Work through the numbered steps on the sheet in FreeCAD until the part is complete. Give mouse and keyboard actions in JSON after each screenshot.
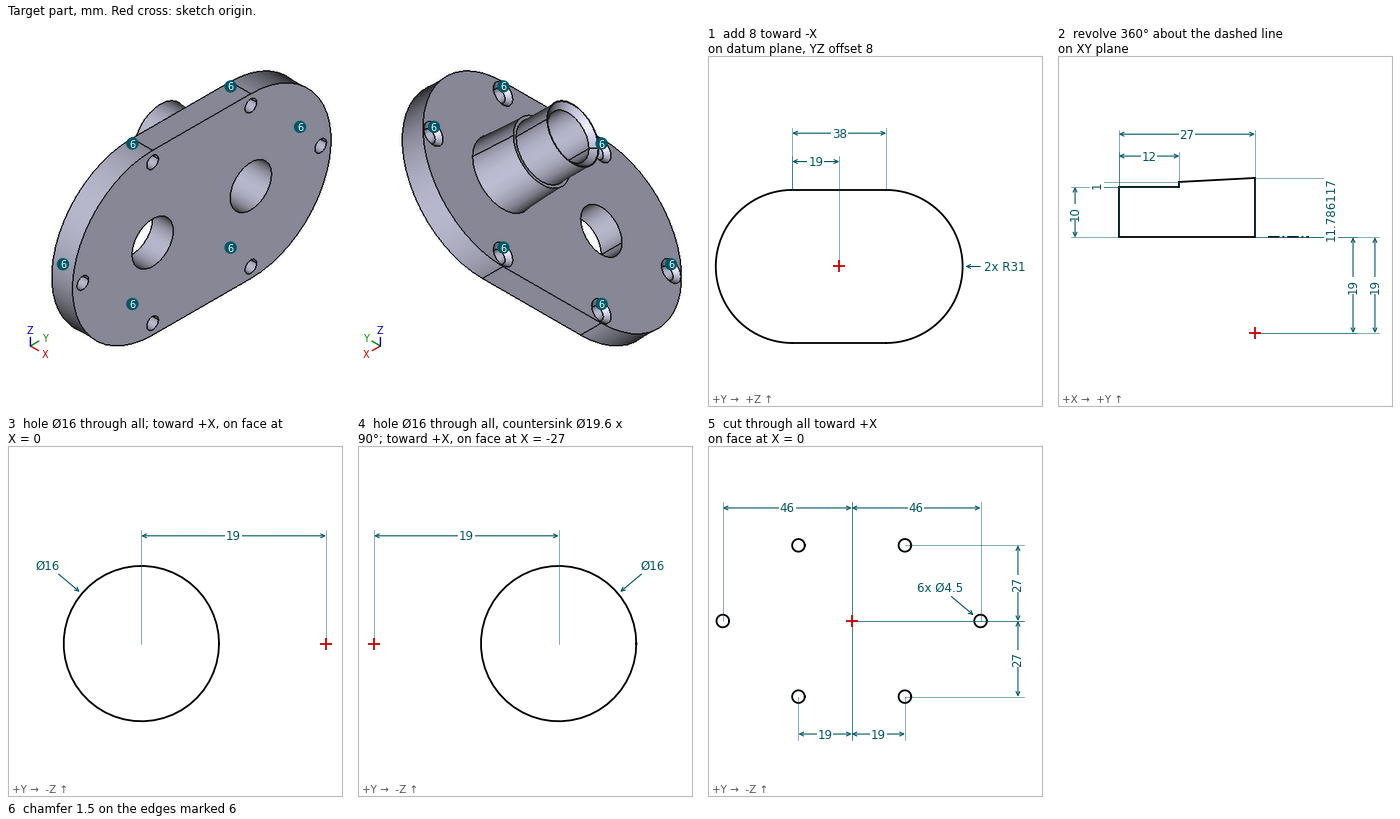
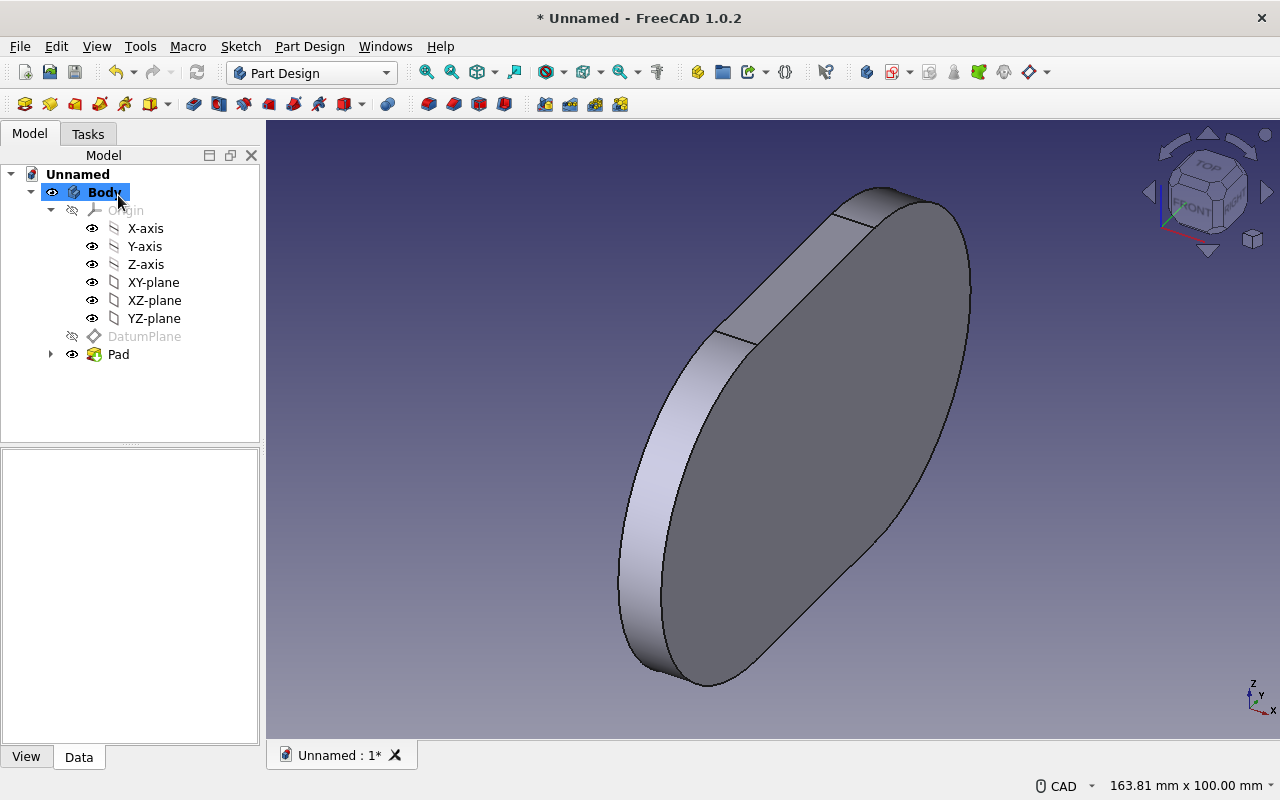
{"action": "key", "text": "v f"}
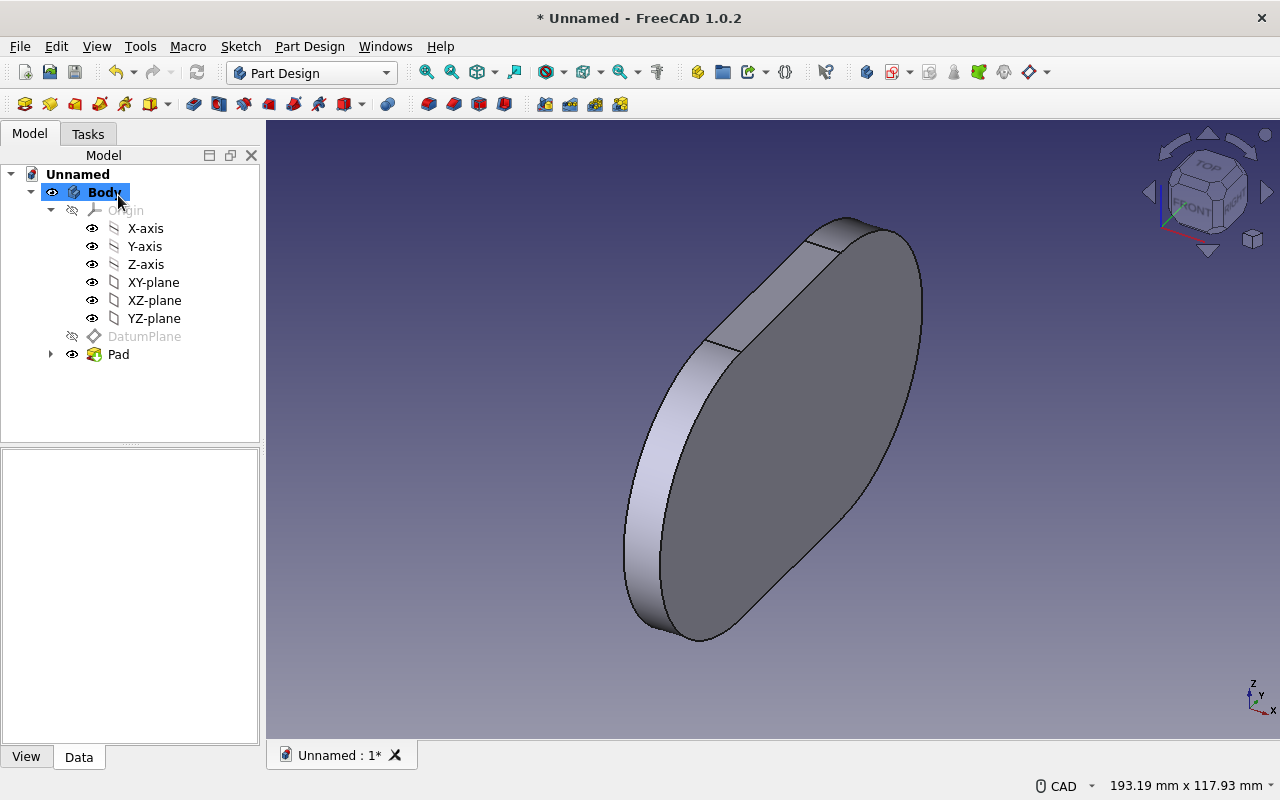
{"action": "left_click", "coordinate": [892, 72]}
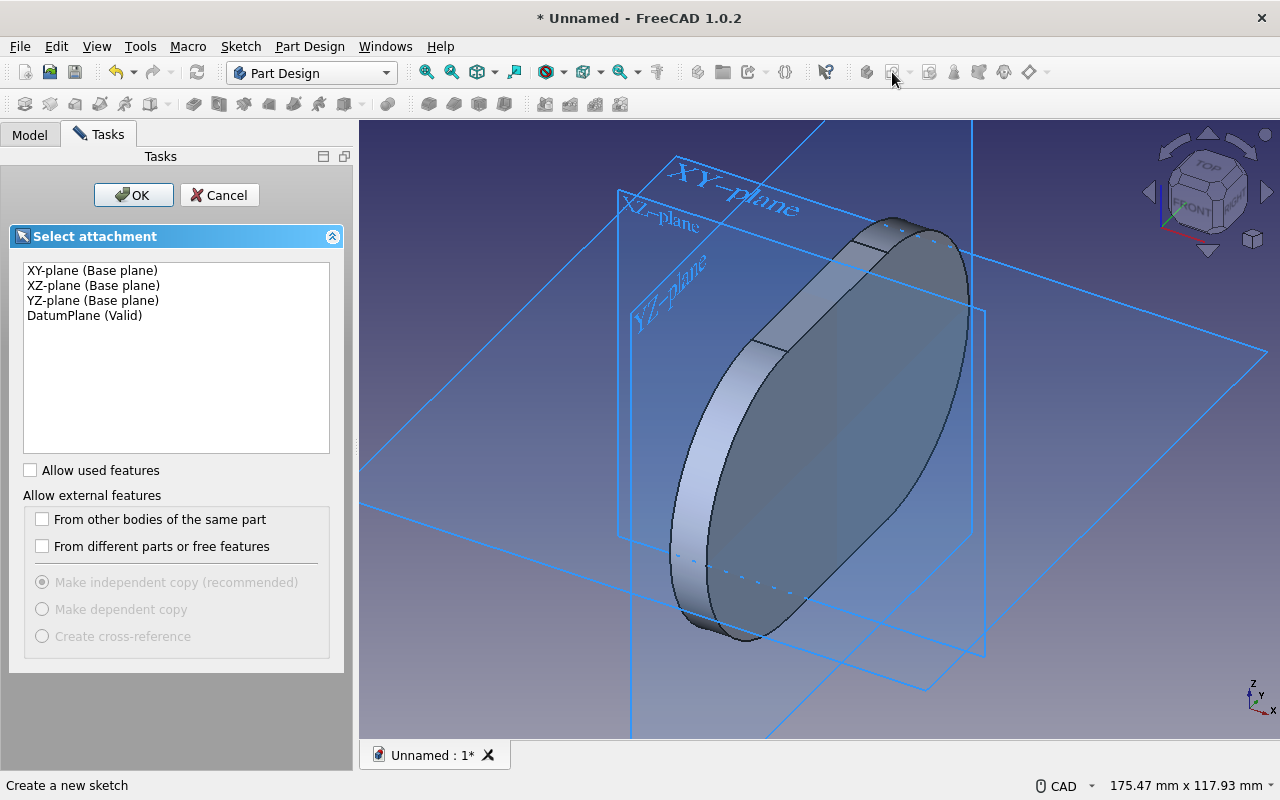
{"action": "left_click", "coordinate": [84, 270]}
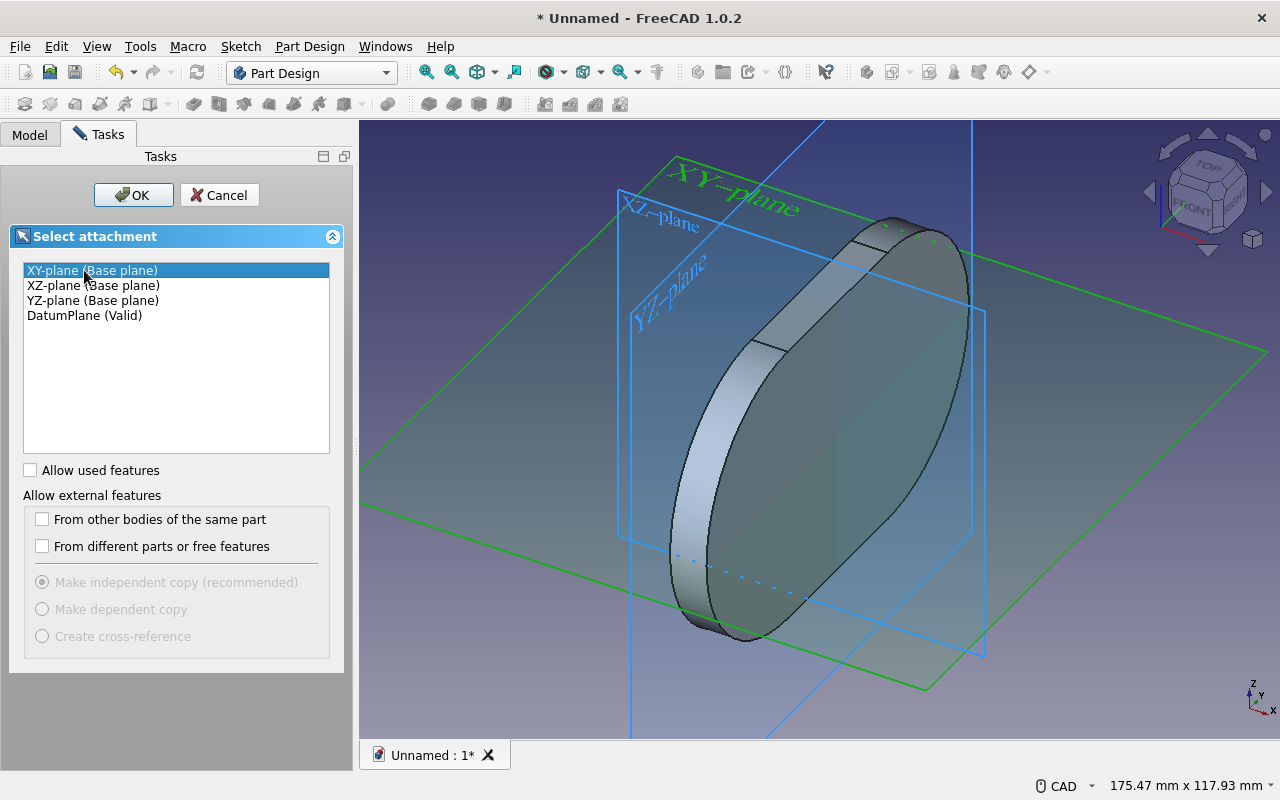
{"action": "left_click", "coordinate": [134, 195]}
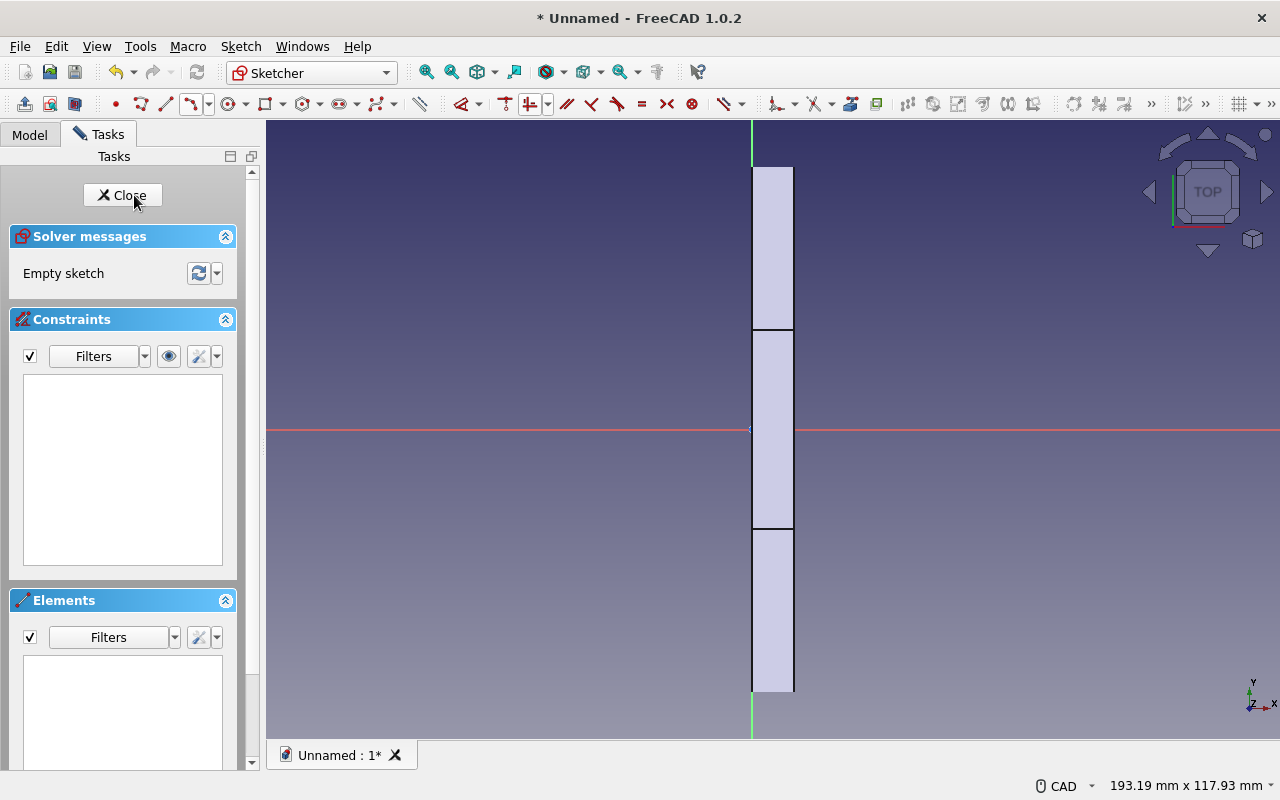
{"action": "key", "text": "q s"}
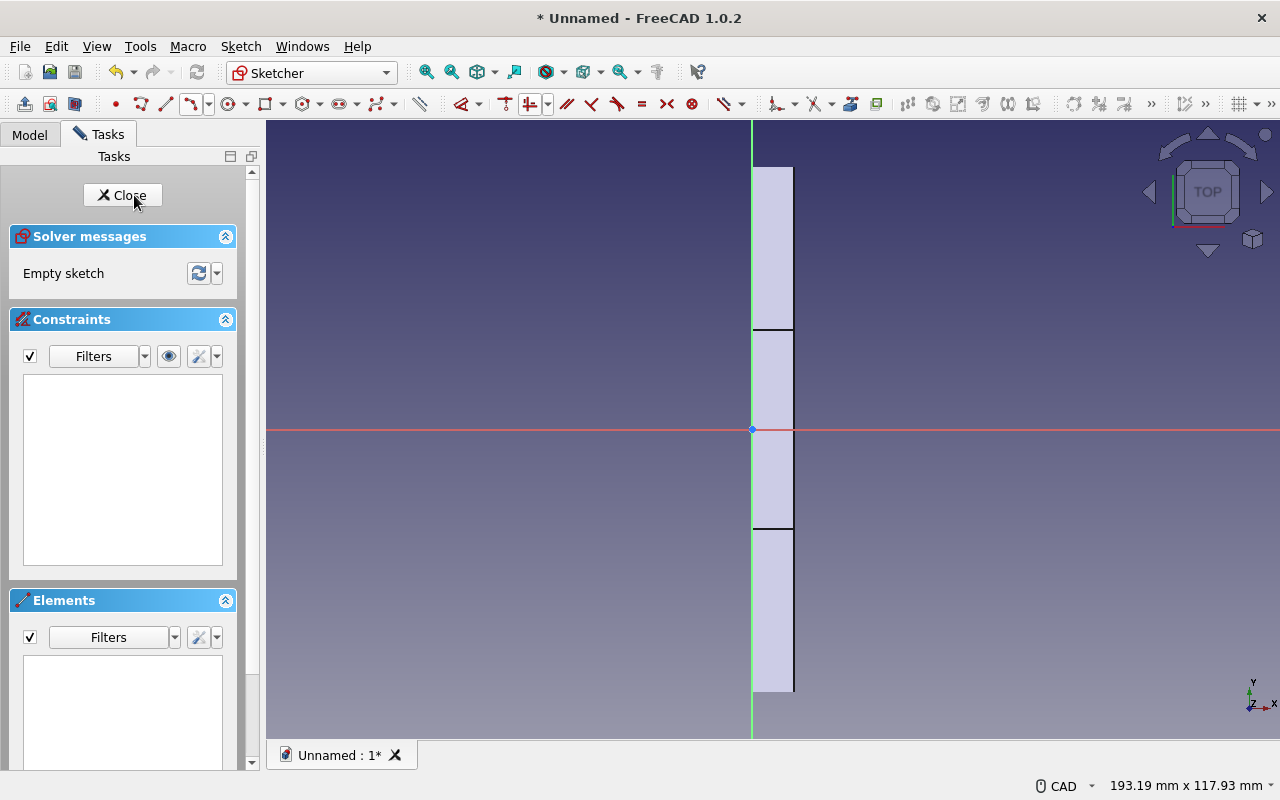
{"action": "scroll", "coordinate": [714, 283], "scroll_direction": "up", "scroll_amount": 4}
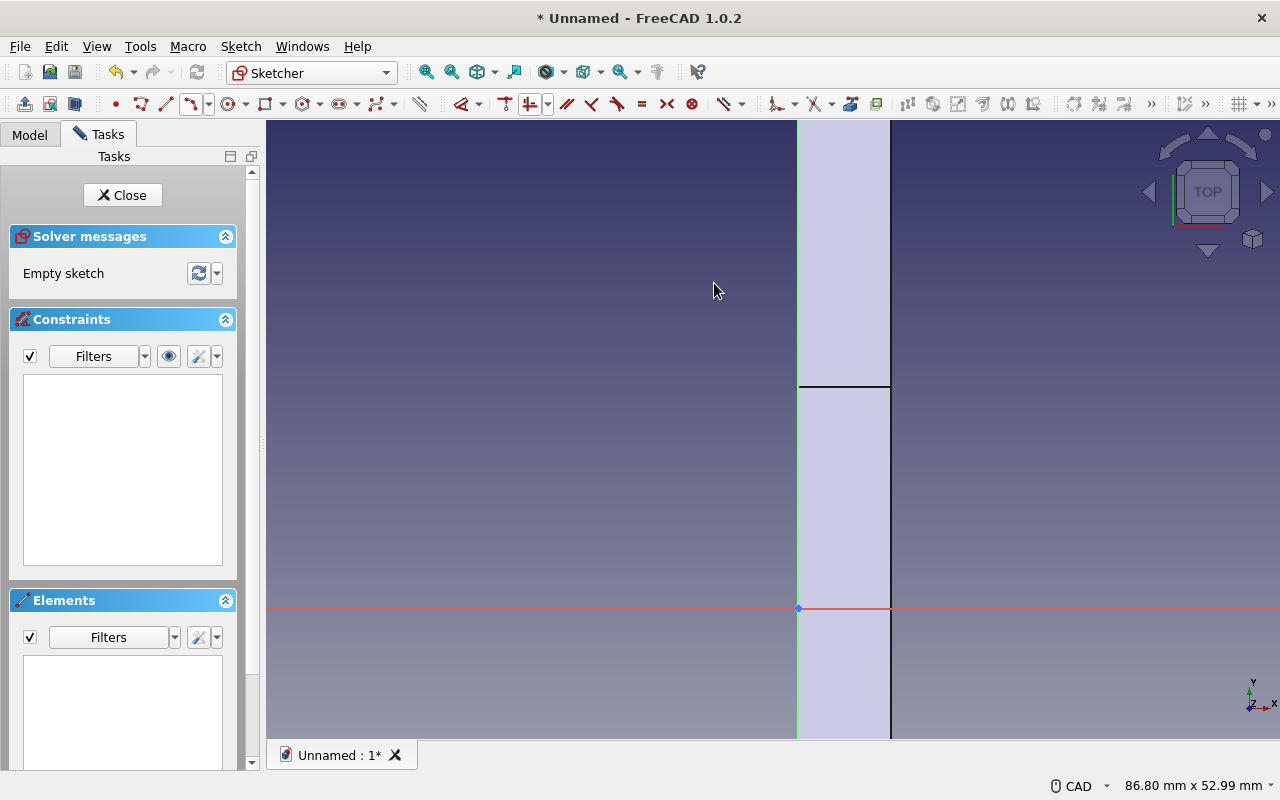
{"action": "key", "text": "g m"}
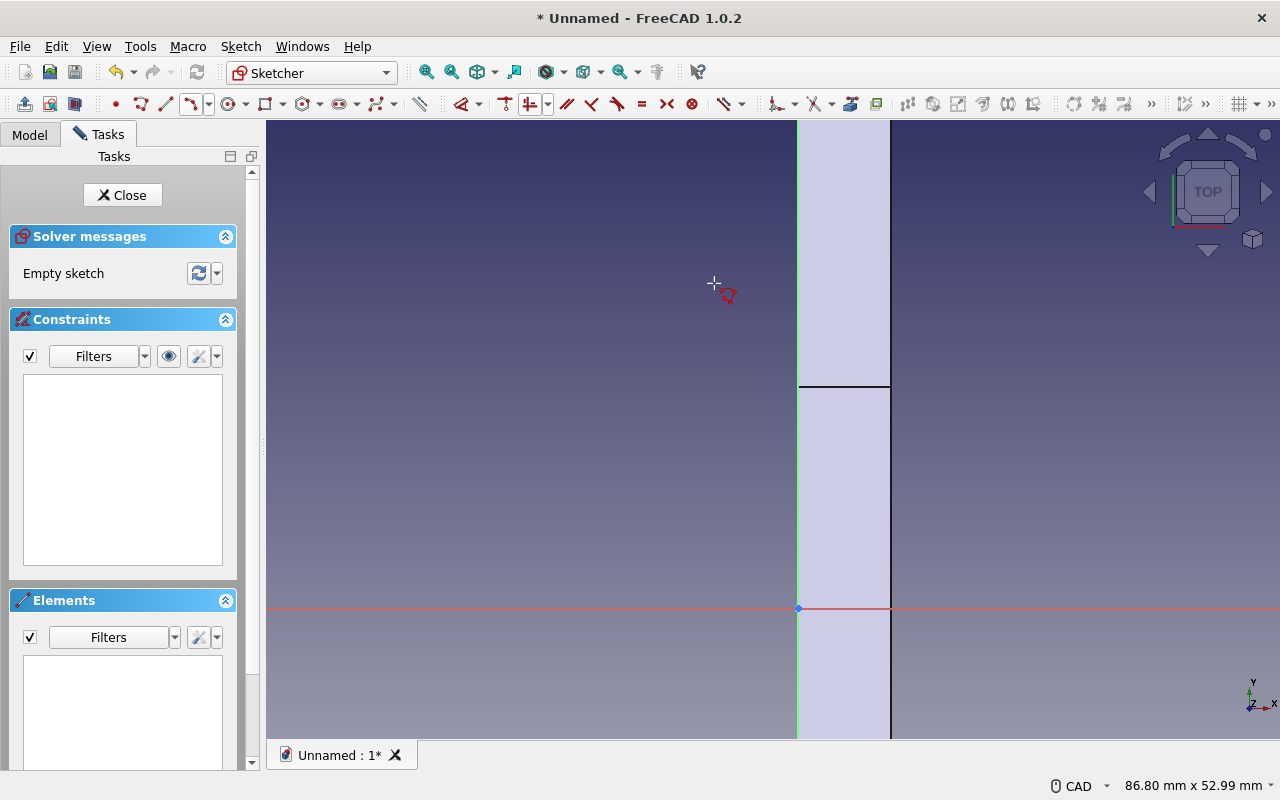
{"action": "left_click", "coordinate": [798, 387]}
{"action": "left_click", "coordinate": [789, 249]}
{"action": "left_click", "coordinate": [623, 258]}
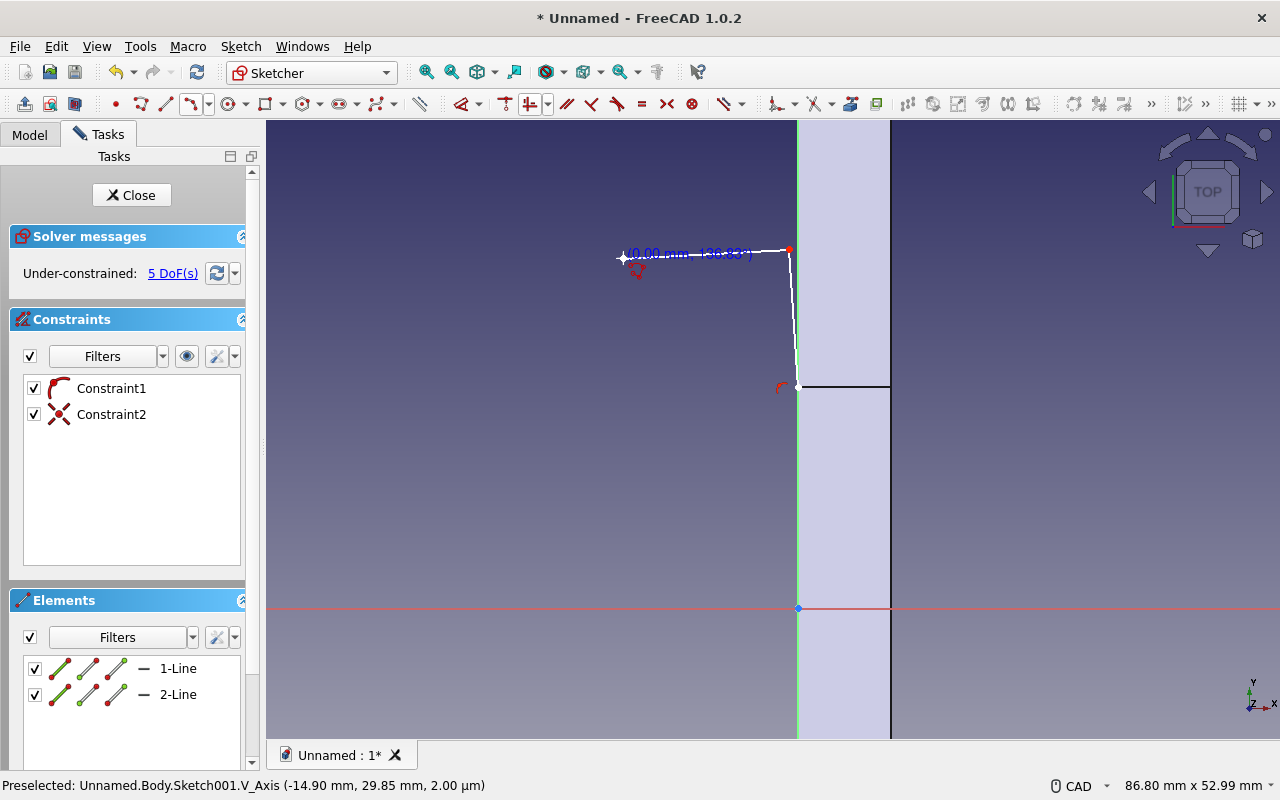
{"action": "scroll", "coordinate": [623, 270], "scroll_direction": "up", "scroll_amount": 2}